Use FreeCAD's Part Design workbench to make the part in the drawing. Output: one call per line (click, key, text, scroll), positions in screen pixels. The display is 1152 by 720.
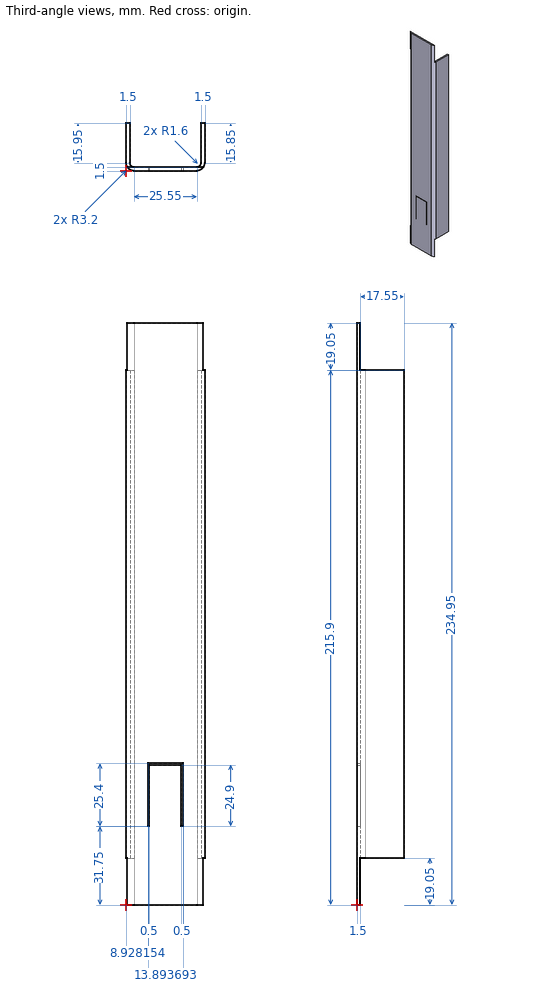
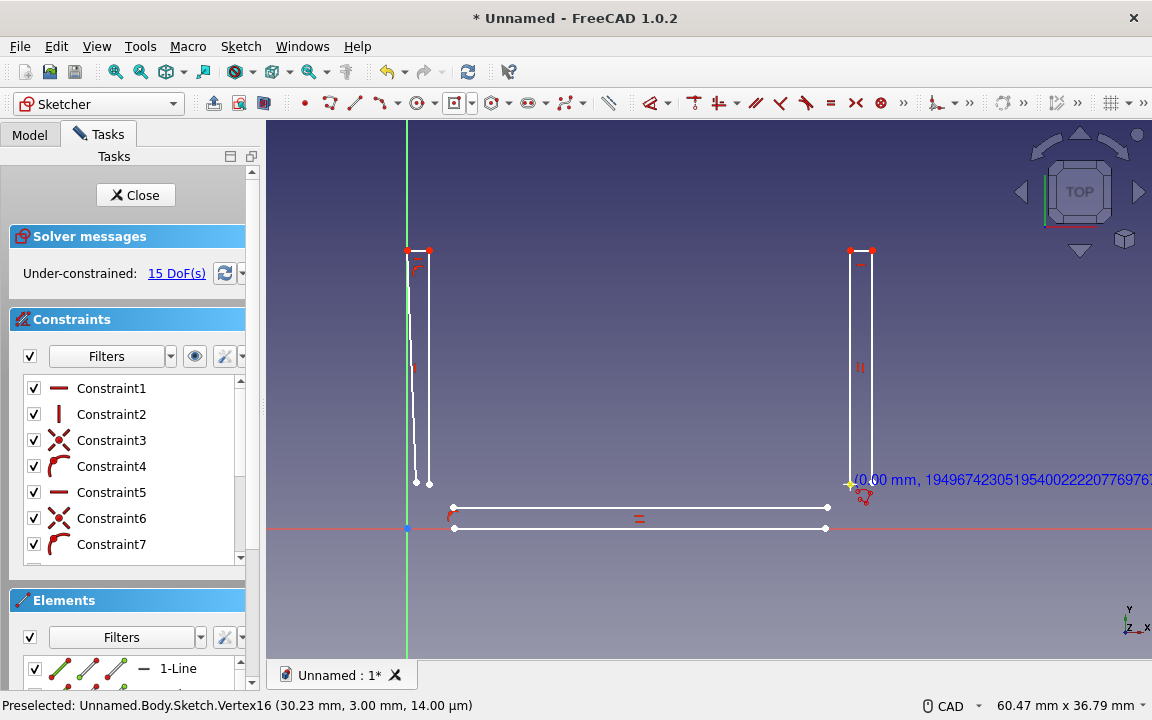
click(380, 104)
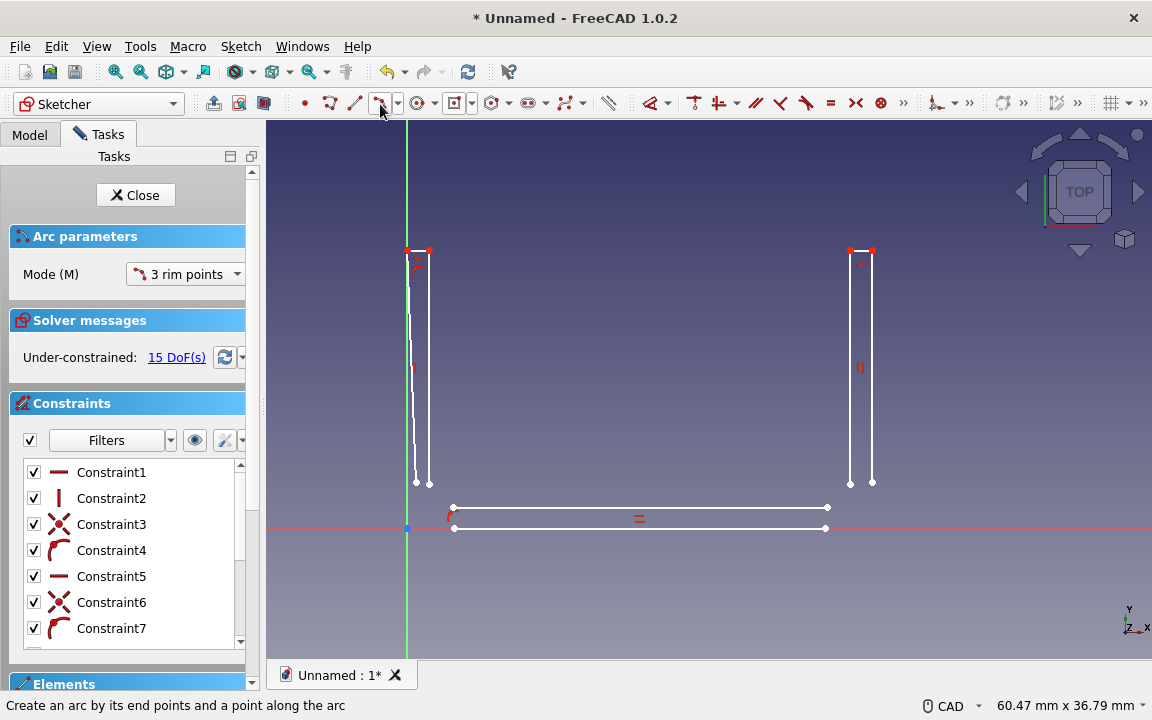
click(453, 508)
click(429, 485)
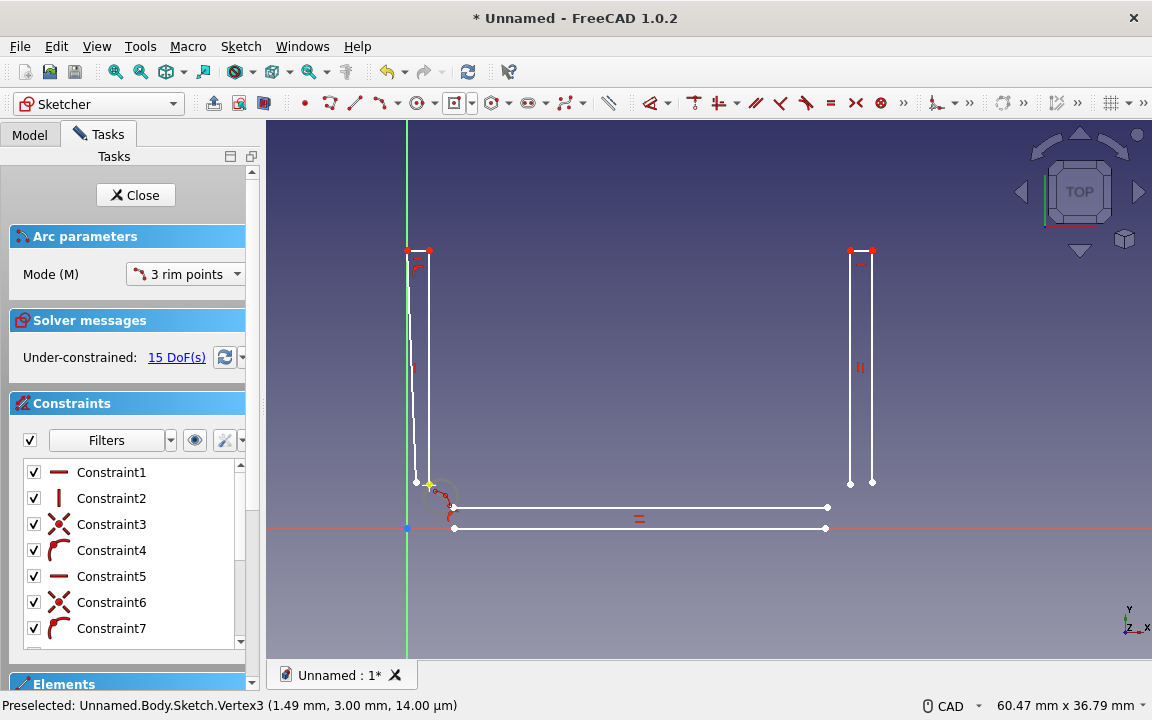
scroll(436, 500, up, 5)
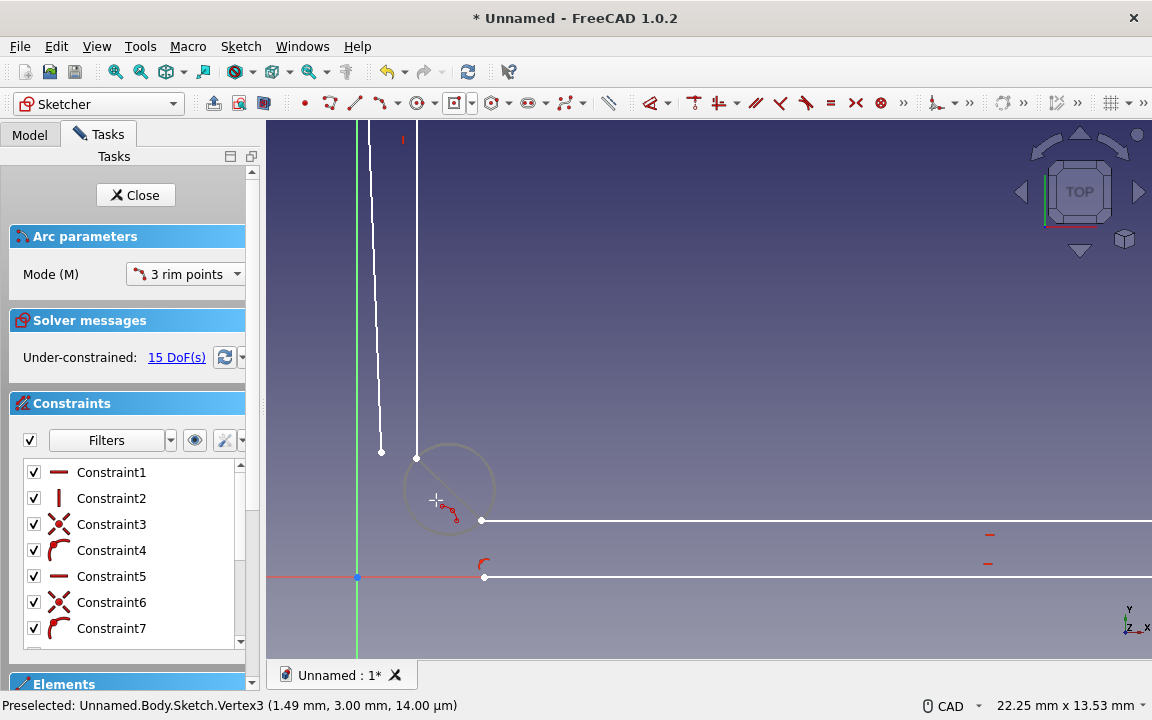
click(436, 499)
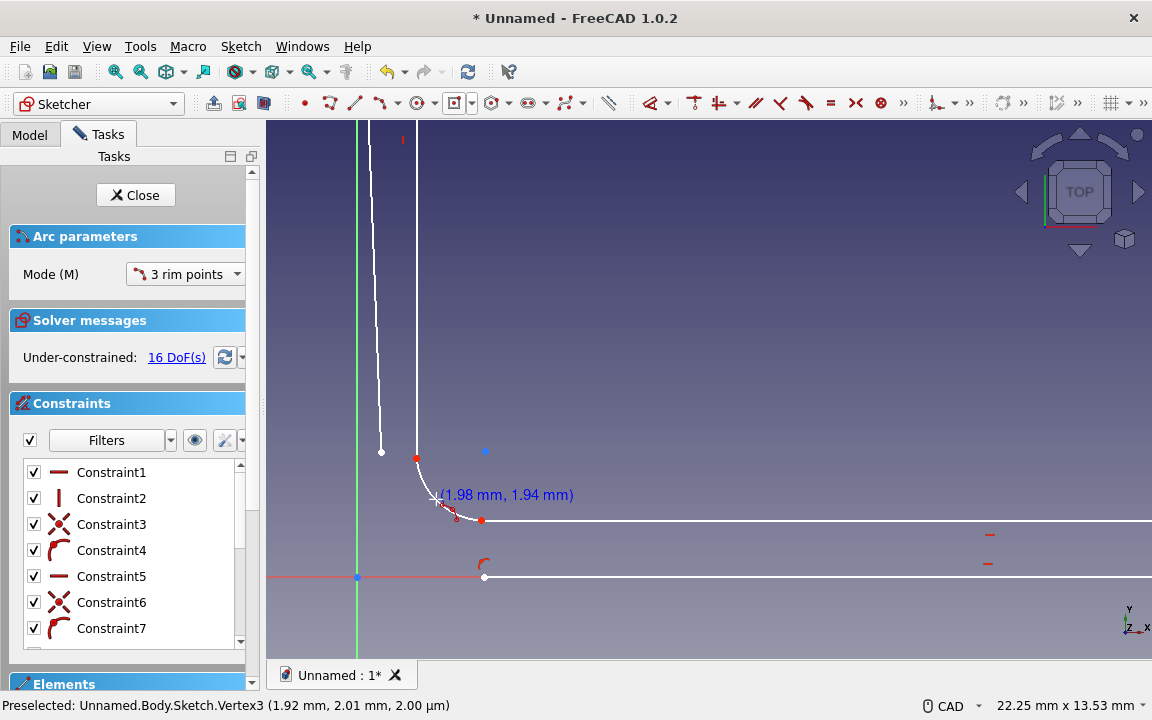
click(381, 453)
click(485, 577)
click(394, 540)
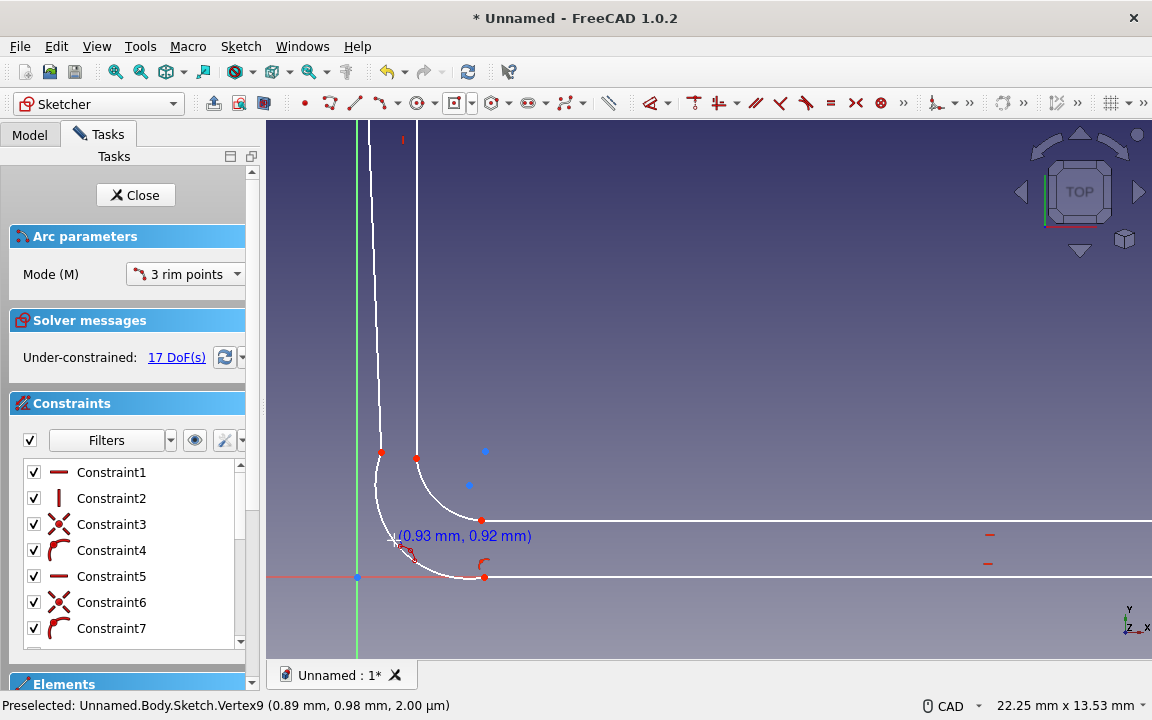
scroll(437, 501, down, 5)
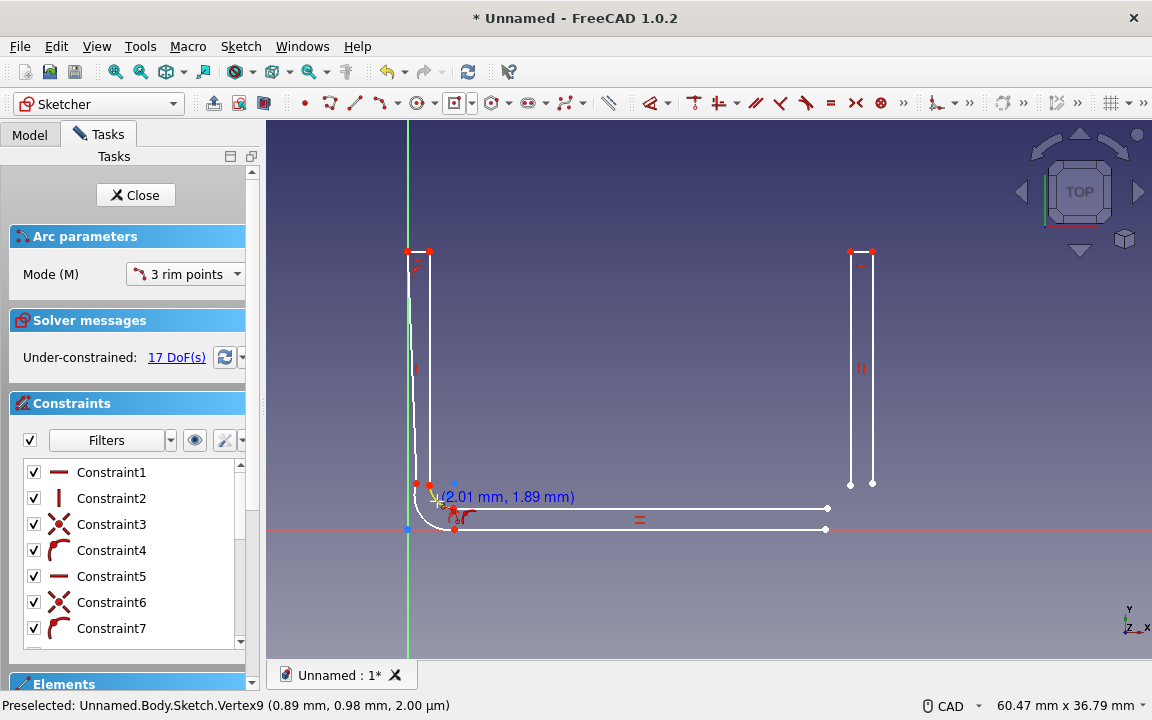
click(826, 530)
click(873, 484)
click(859, 516)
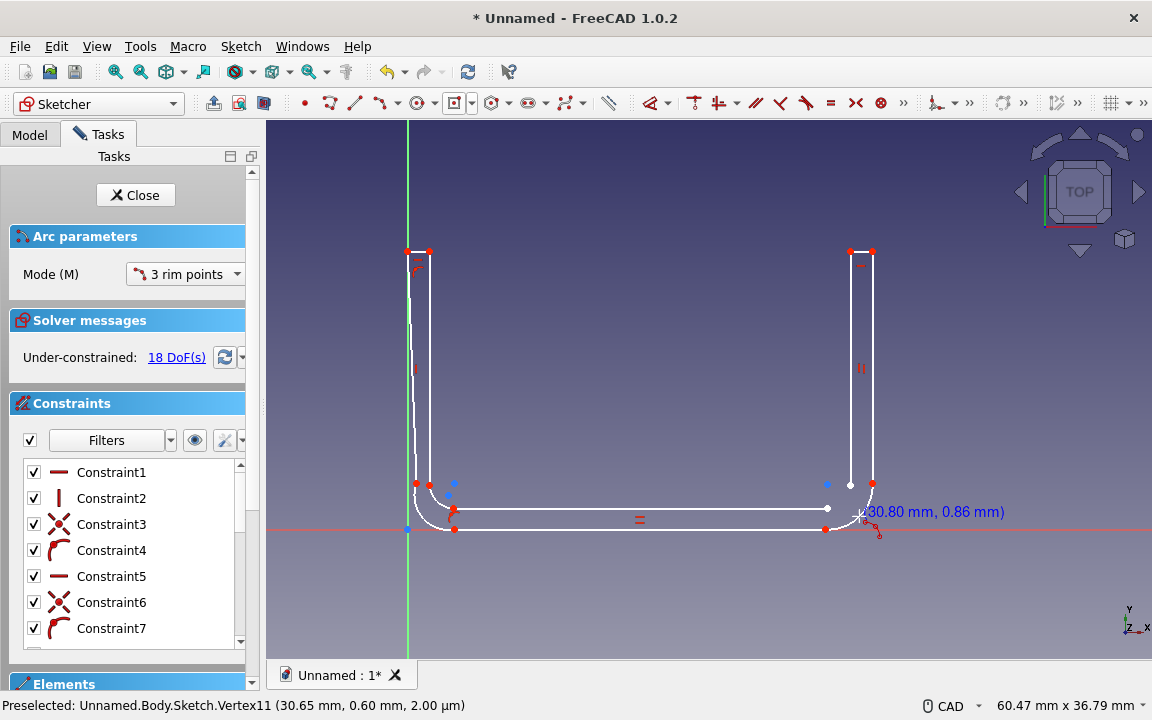
click(851, 486)
click(828, 509)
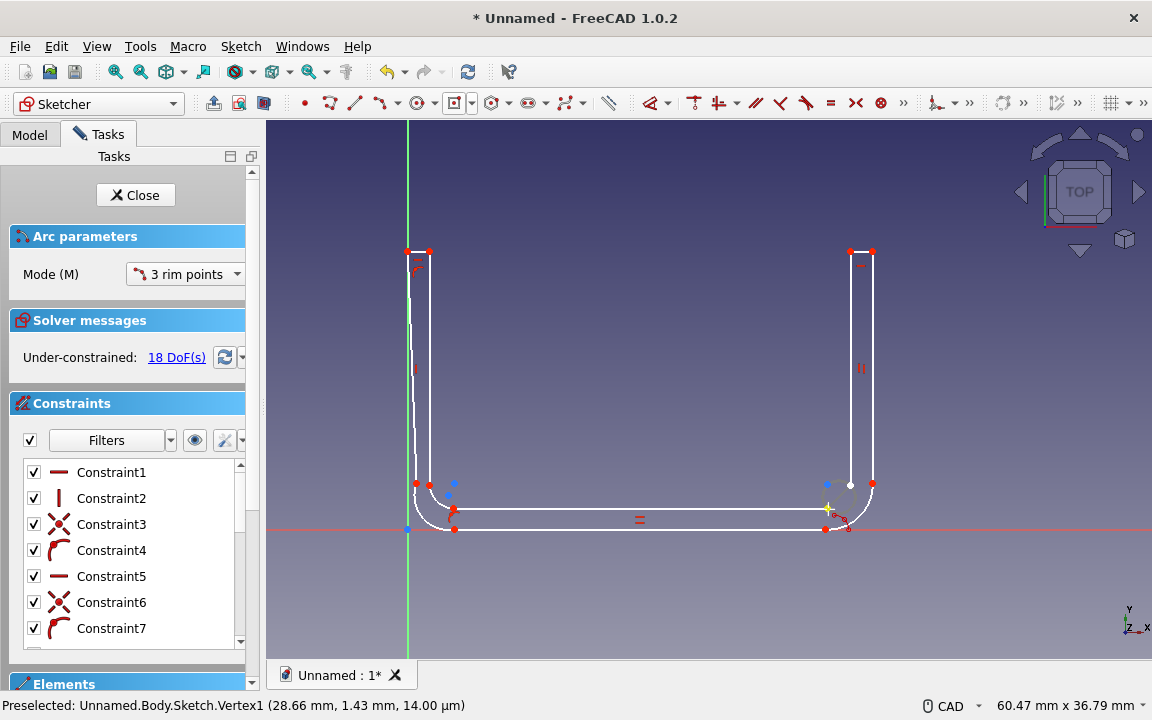
scroll(844, 501, up, 5)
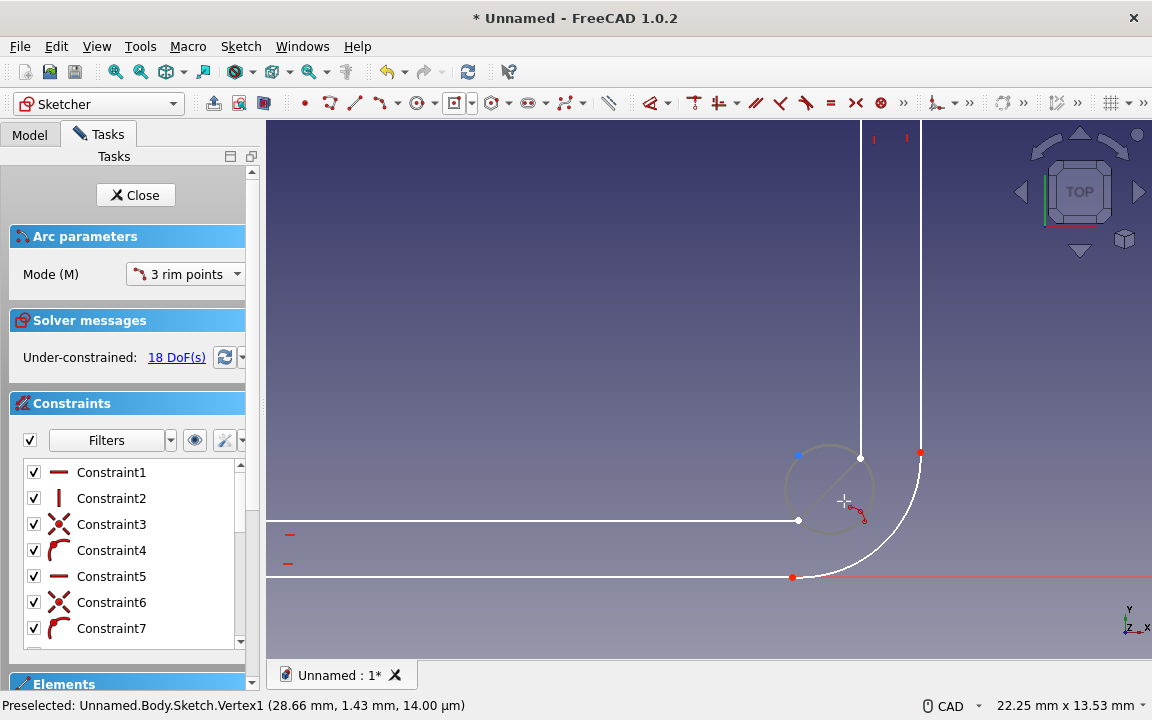
click(843, 499)
key(Escape)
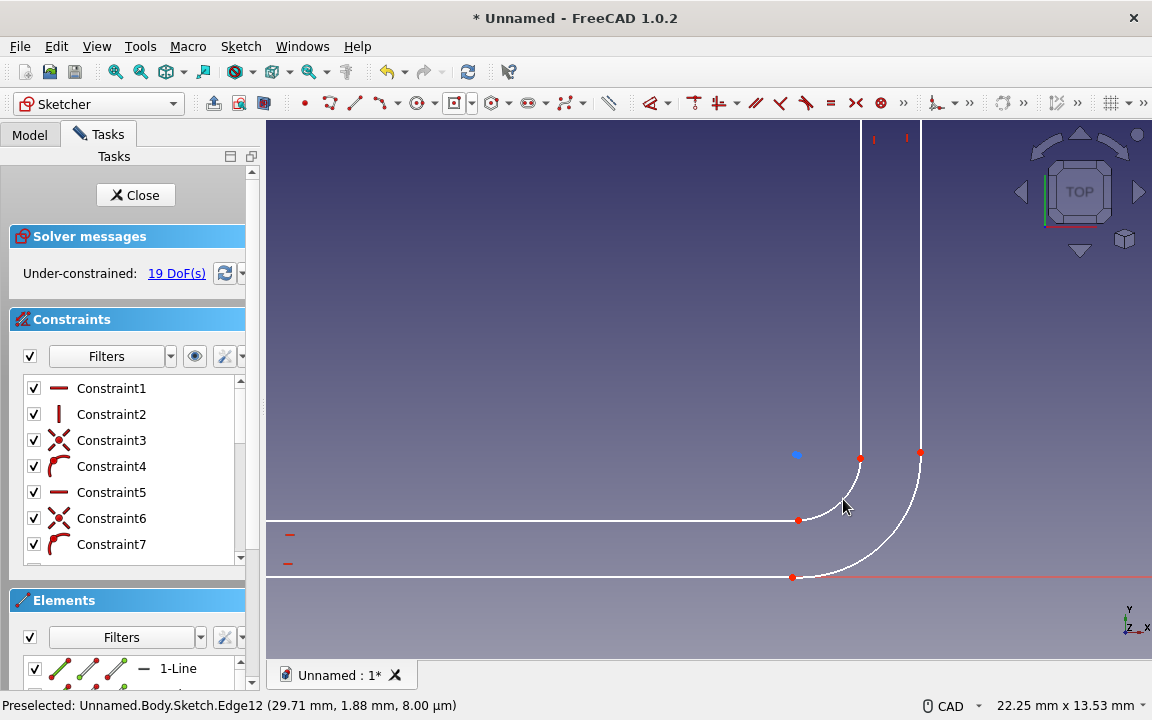
click(493, 521)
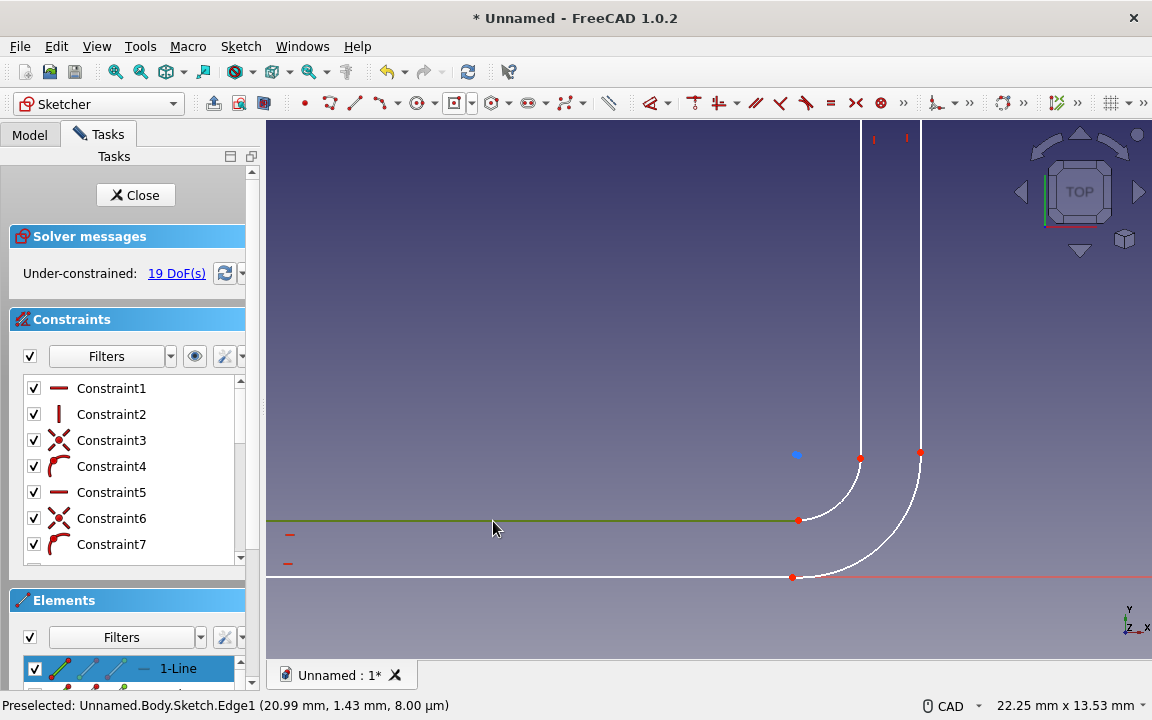
scroll(845, 501, down, 5)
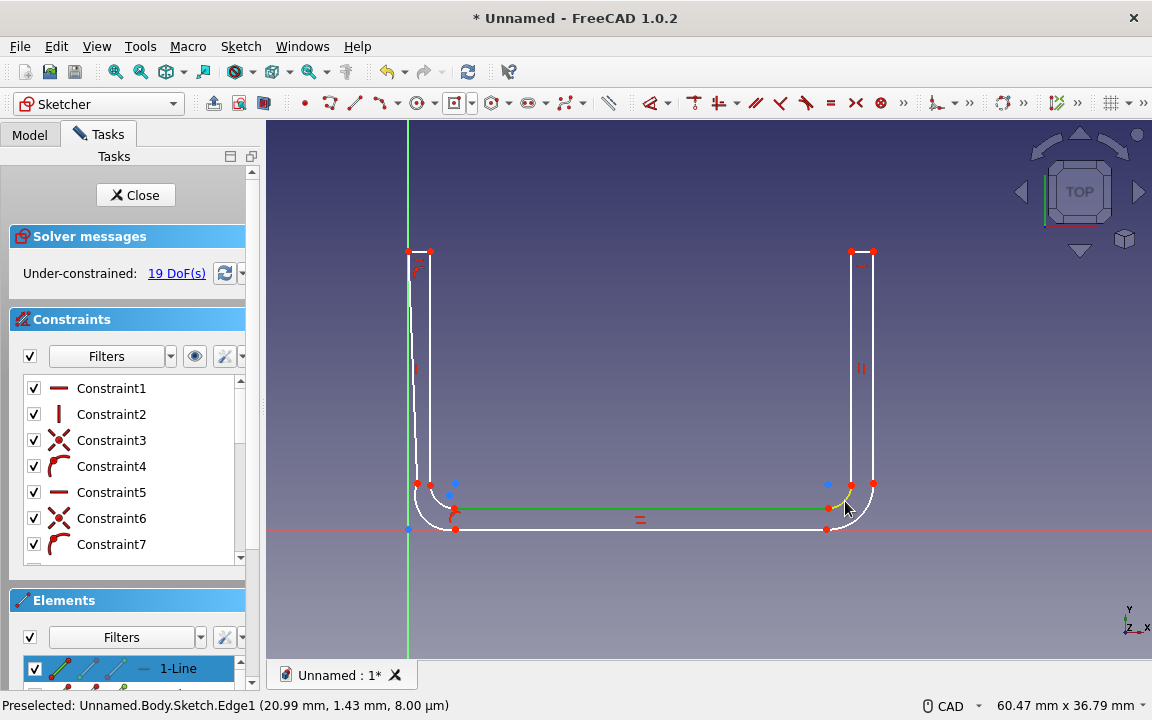
scroll(433, 496, up, 2)